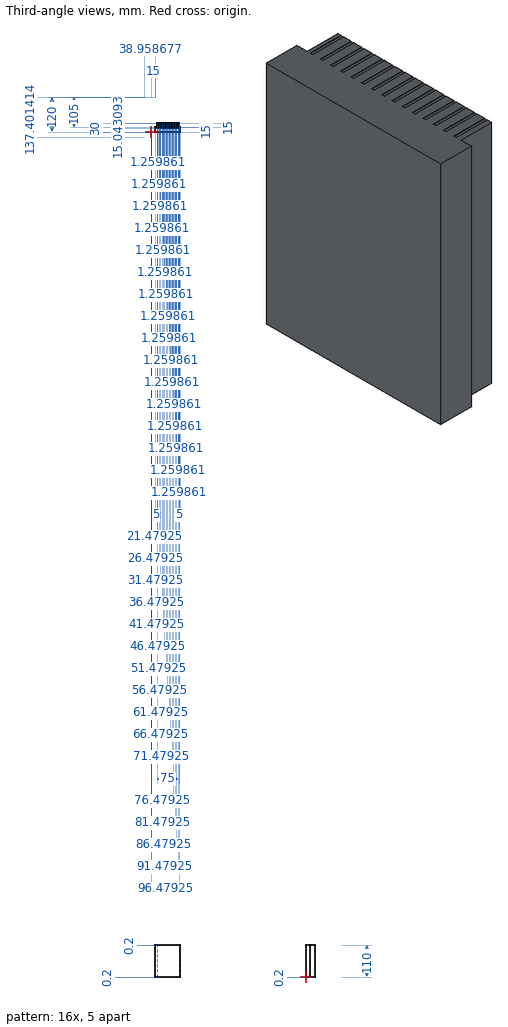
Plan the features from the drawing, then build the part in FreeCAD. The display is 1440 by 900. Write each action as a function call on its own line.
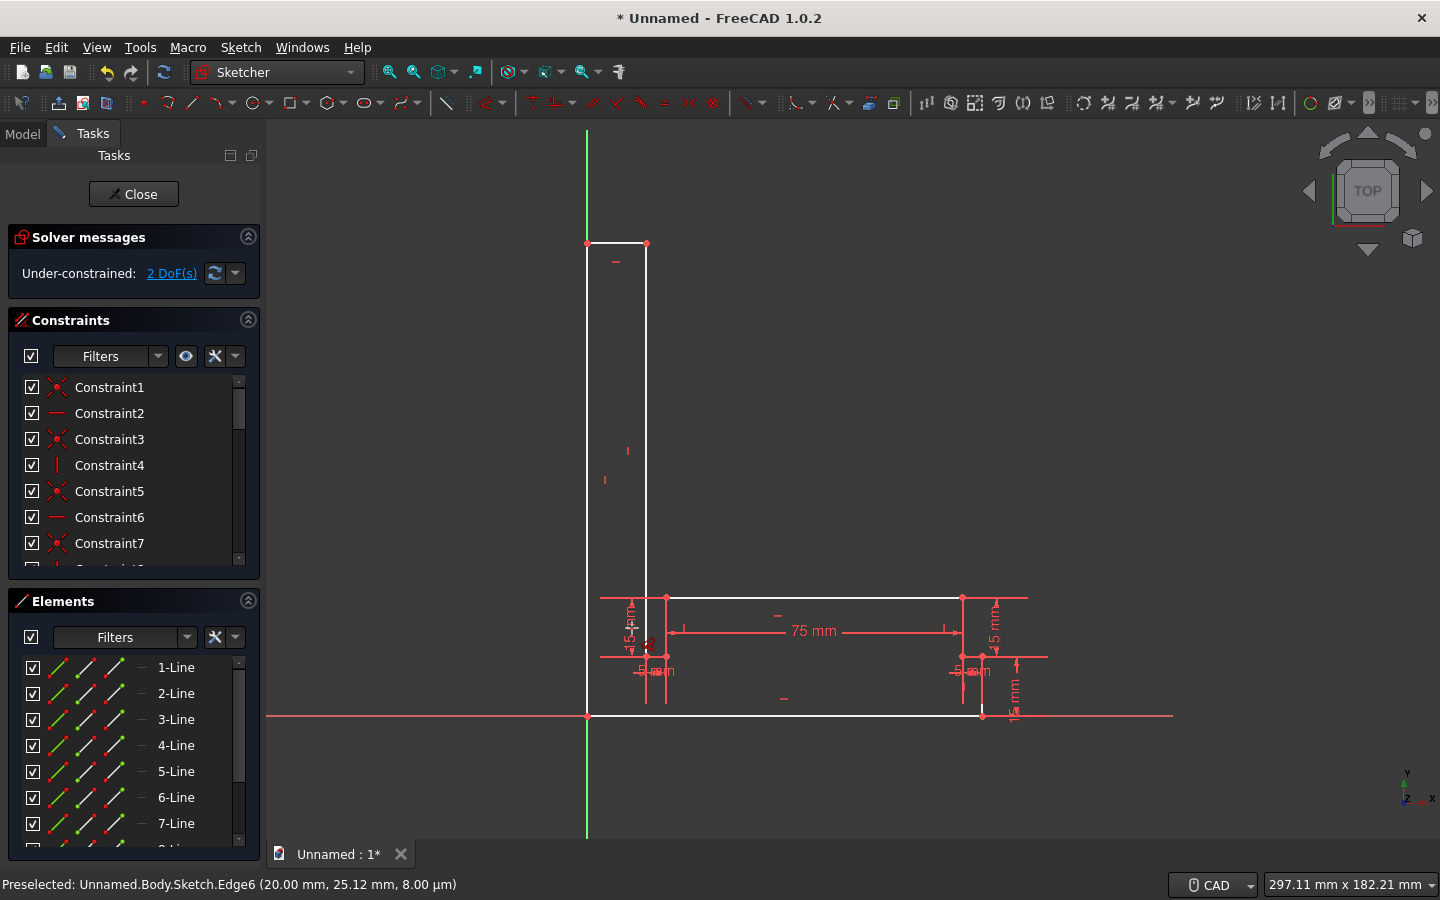
click(629, 243)
click(617, 209)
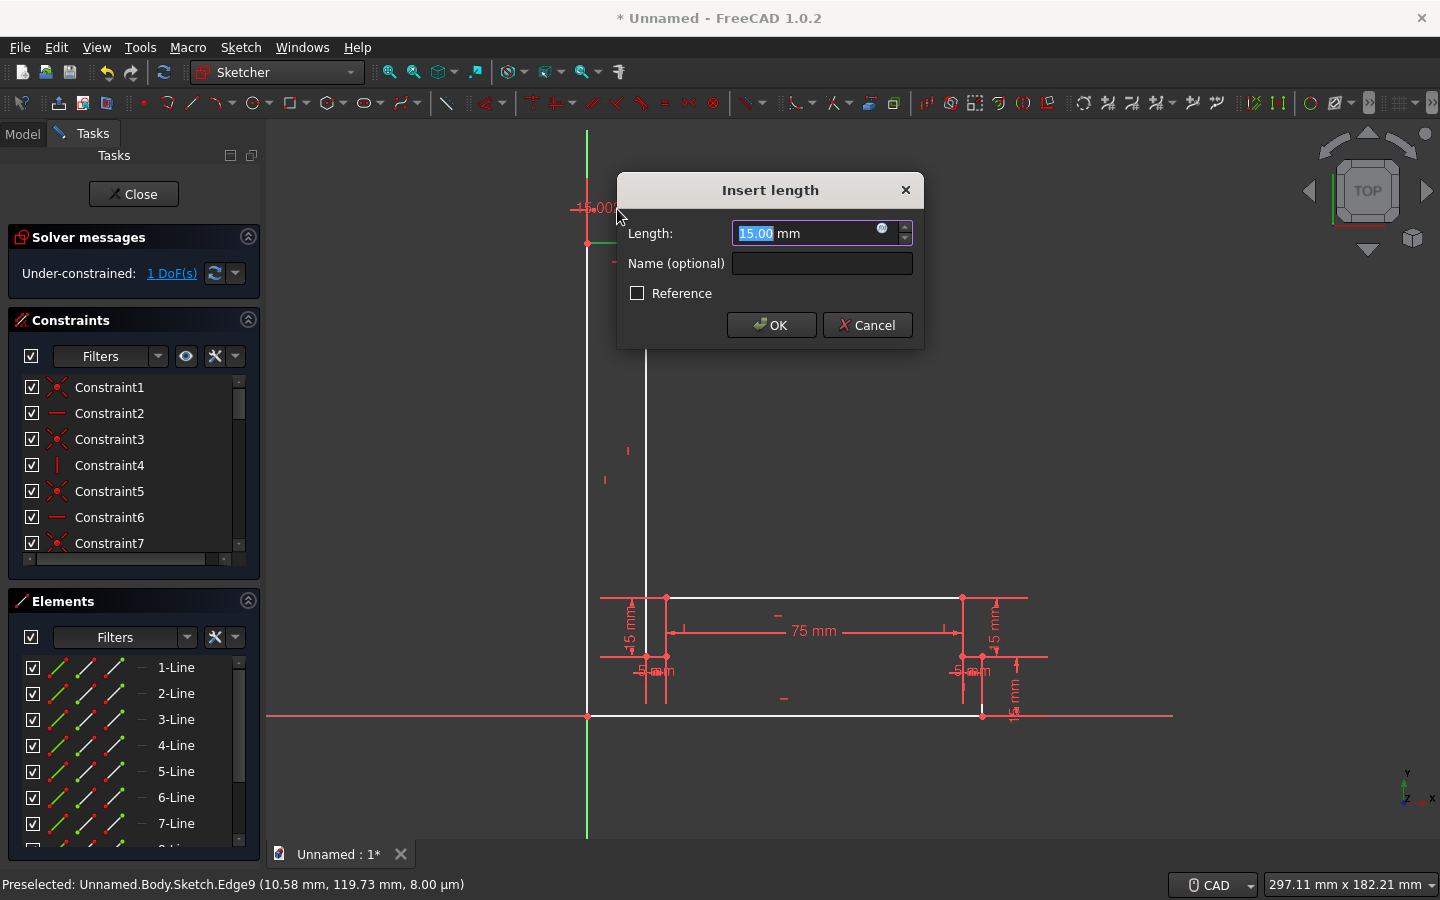
text(15)
key(Return)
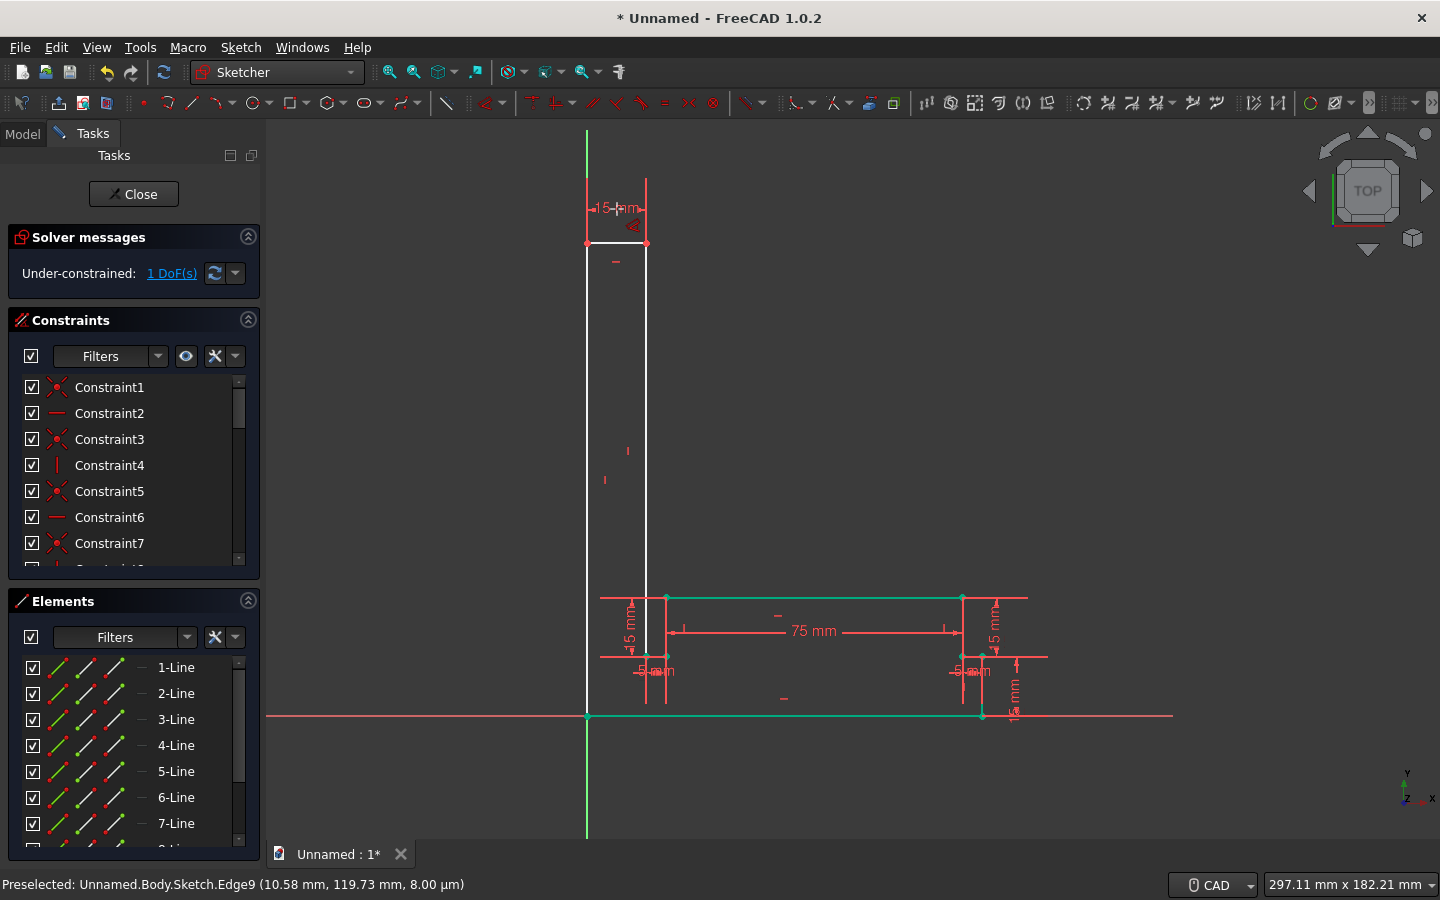
click(646, 533)
click(612, 450)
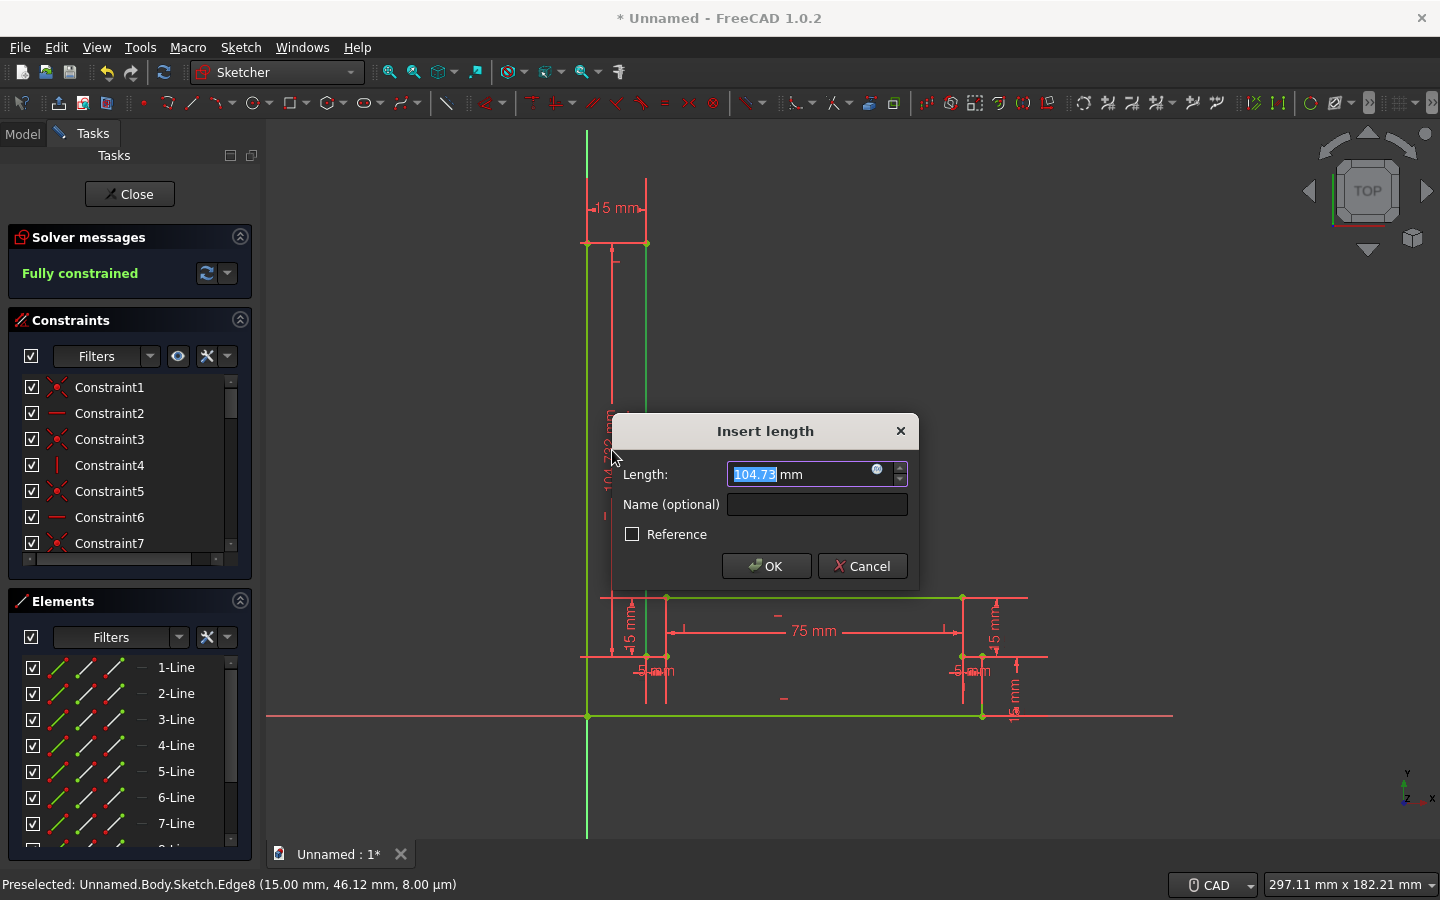
text(105)
key(Return)
key(Escape)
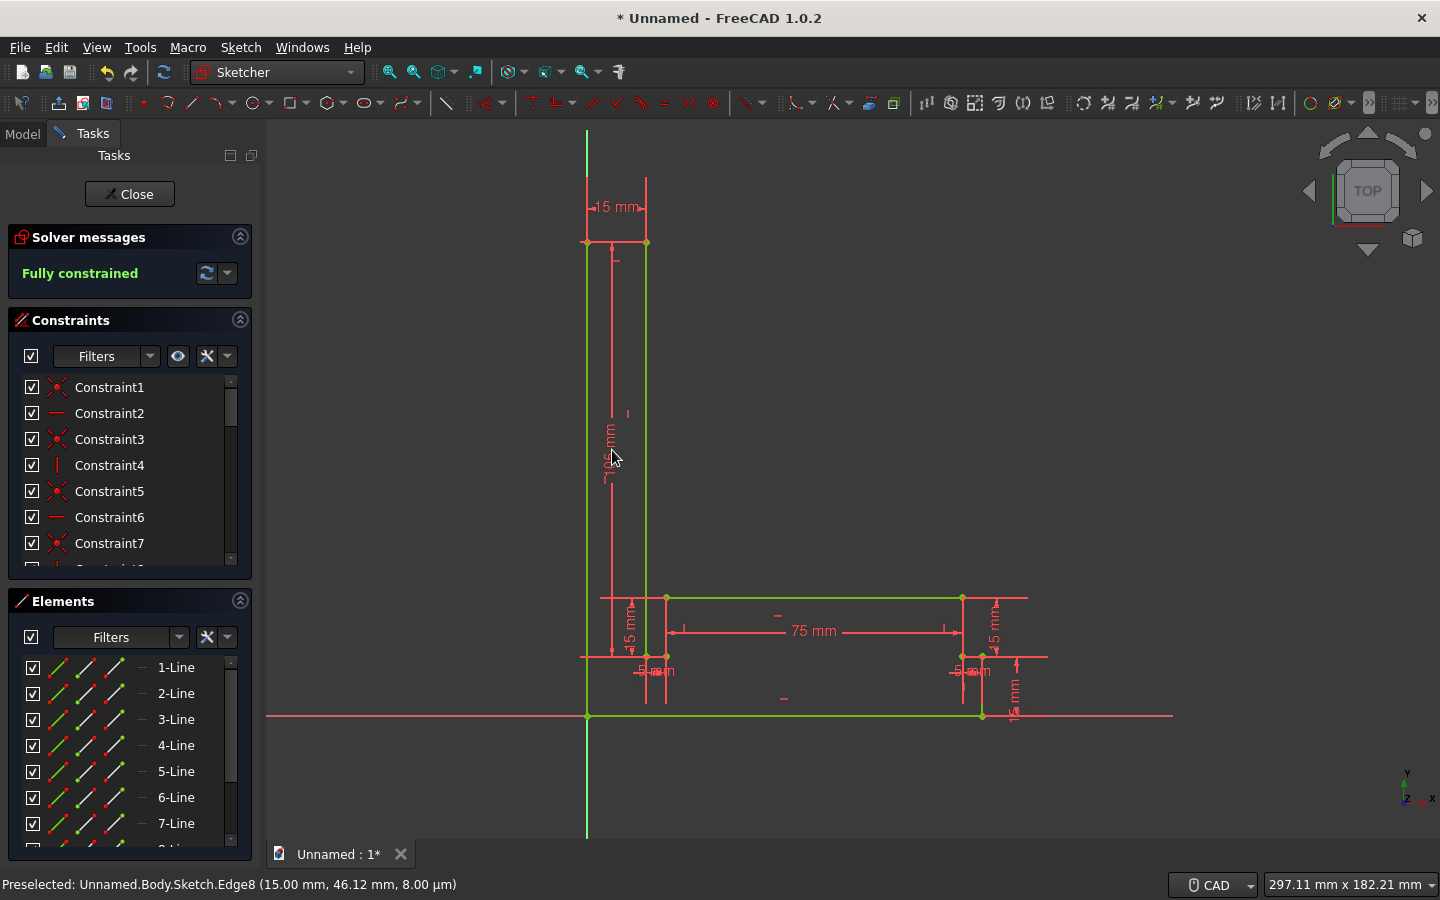
click(130, 194)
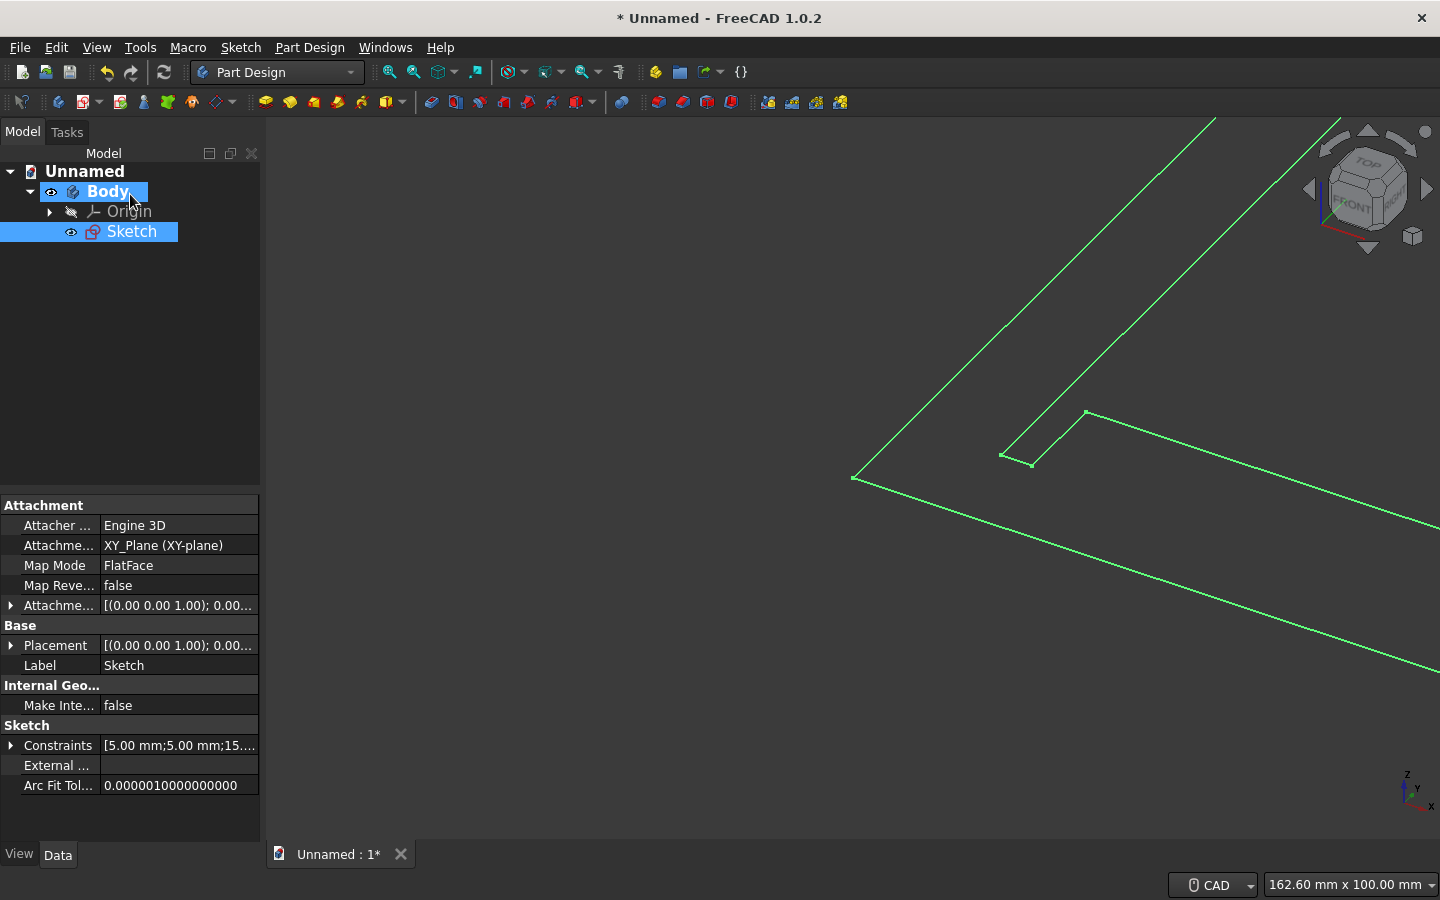
click(266, 102)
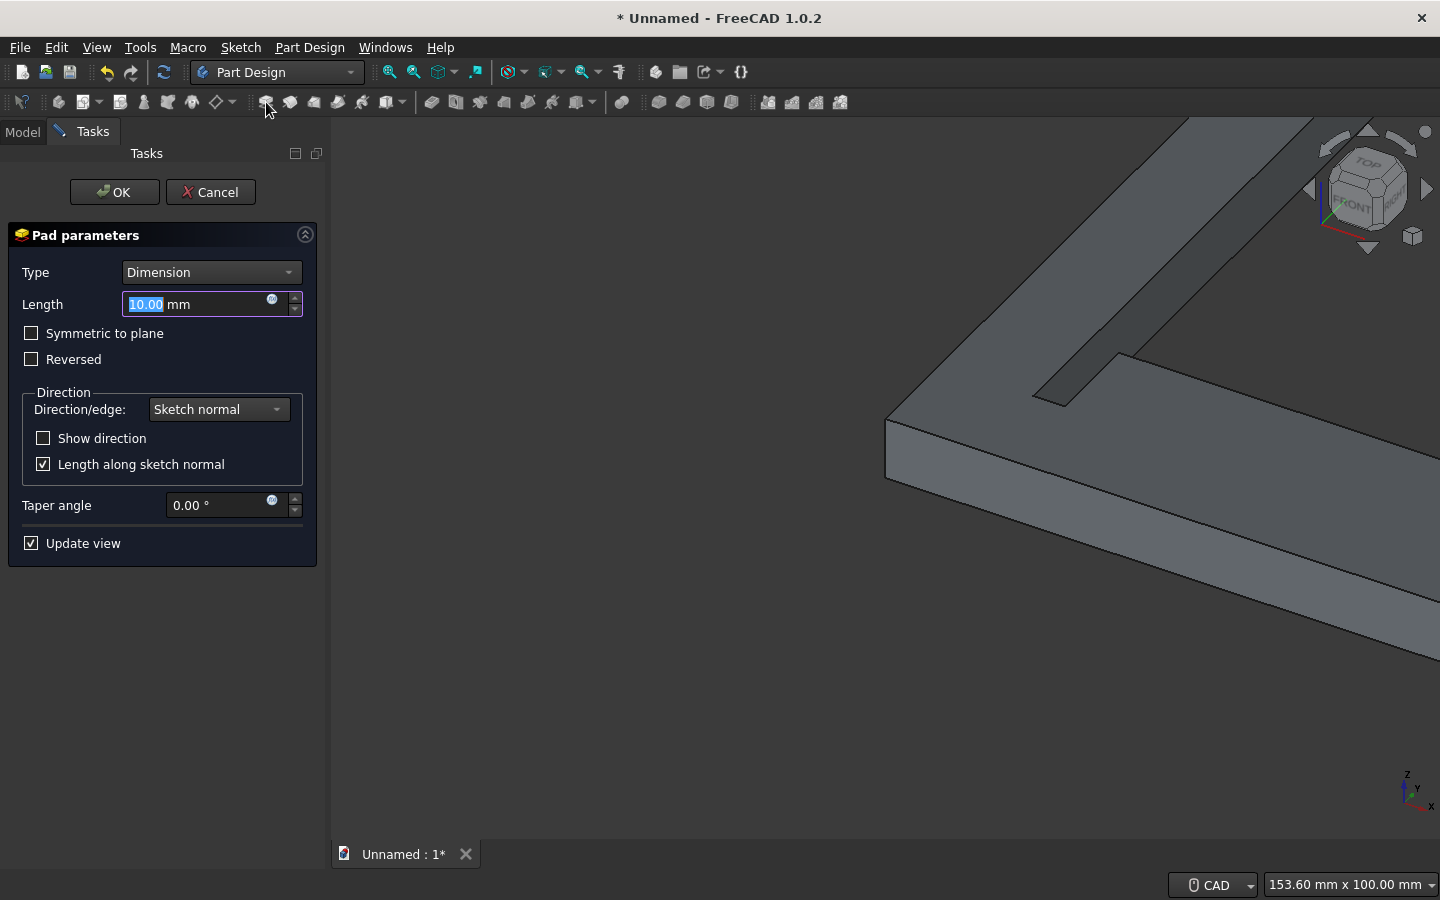
text(110)
key(Tab)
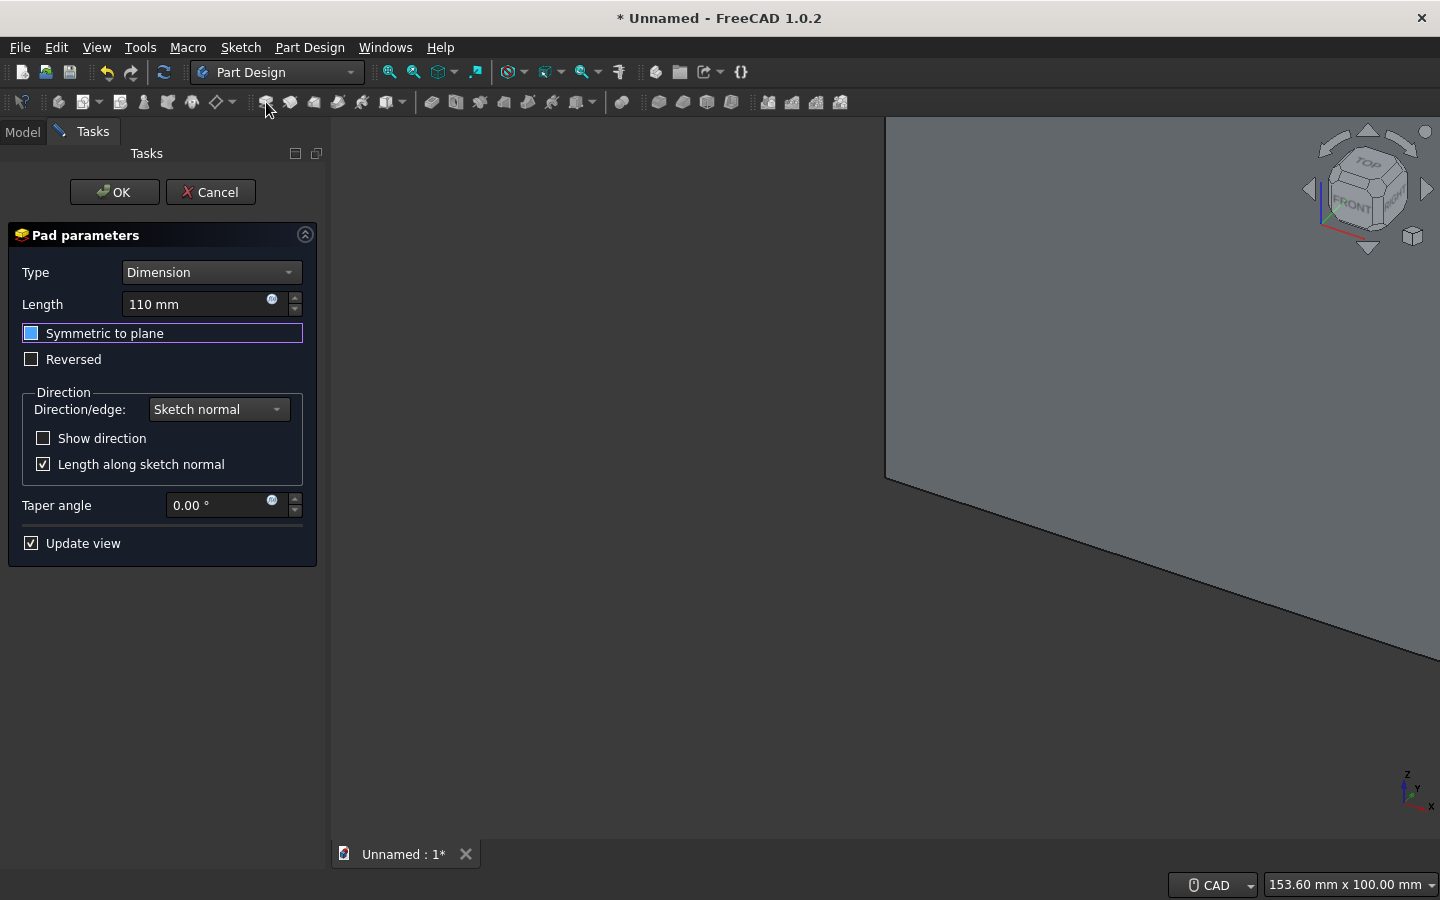
click(115, 192)